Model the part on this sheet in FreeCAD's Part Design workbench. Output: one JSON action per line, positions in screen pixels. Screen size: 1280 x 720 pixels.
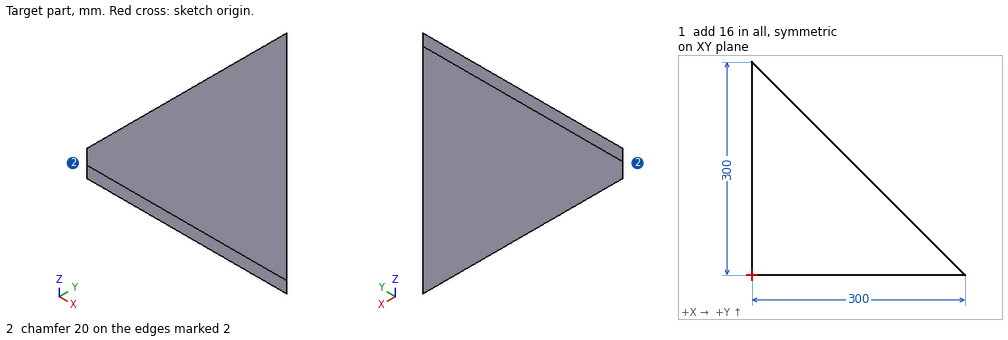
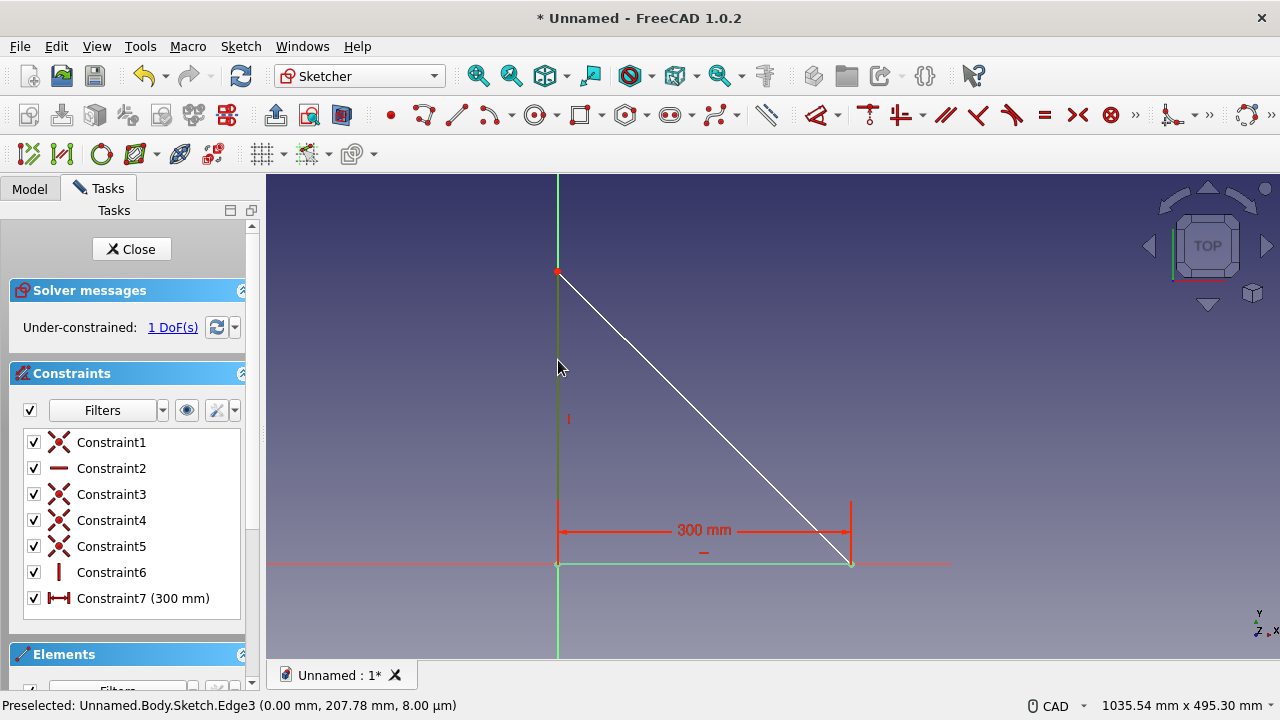
{"action": "key", "text": "i"}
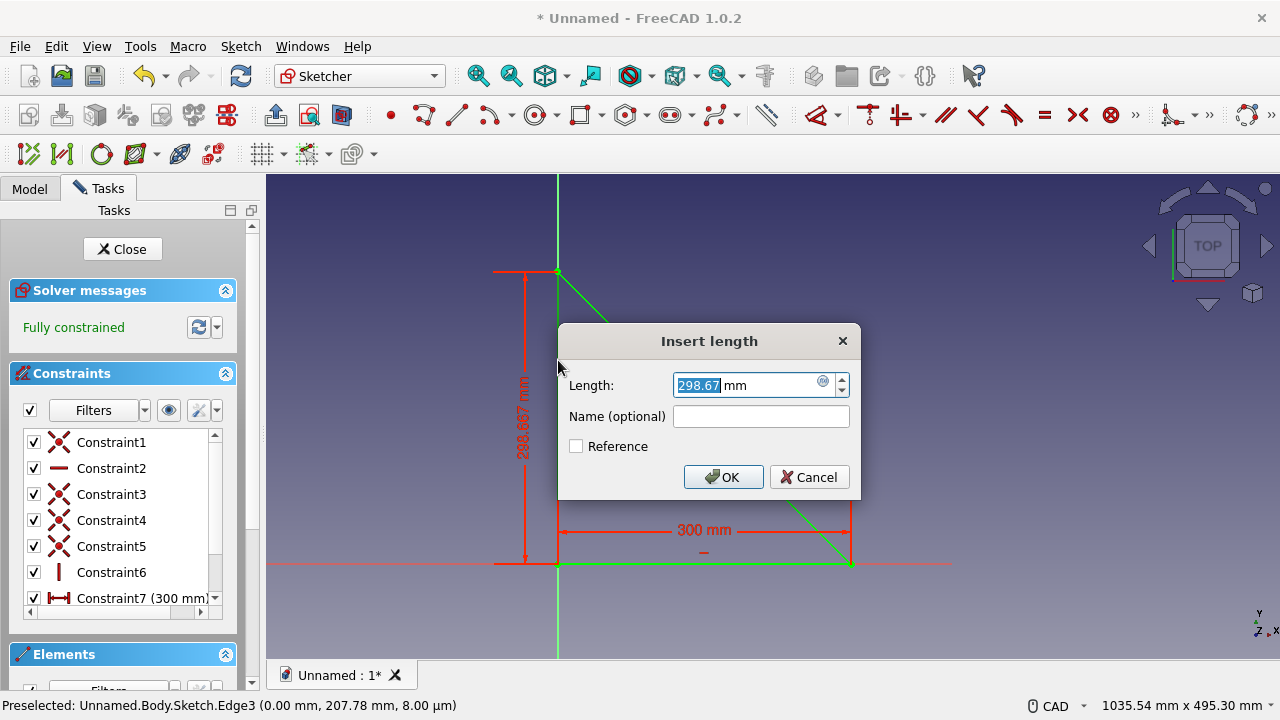
{"action": "type", "text": "300"}
{"action": "key", "text": "Return"}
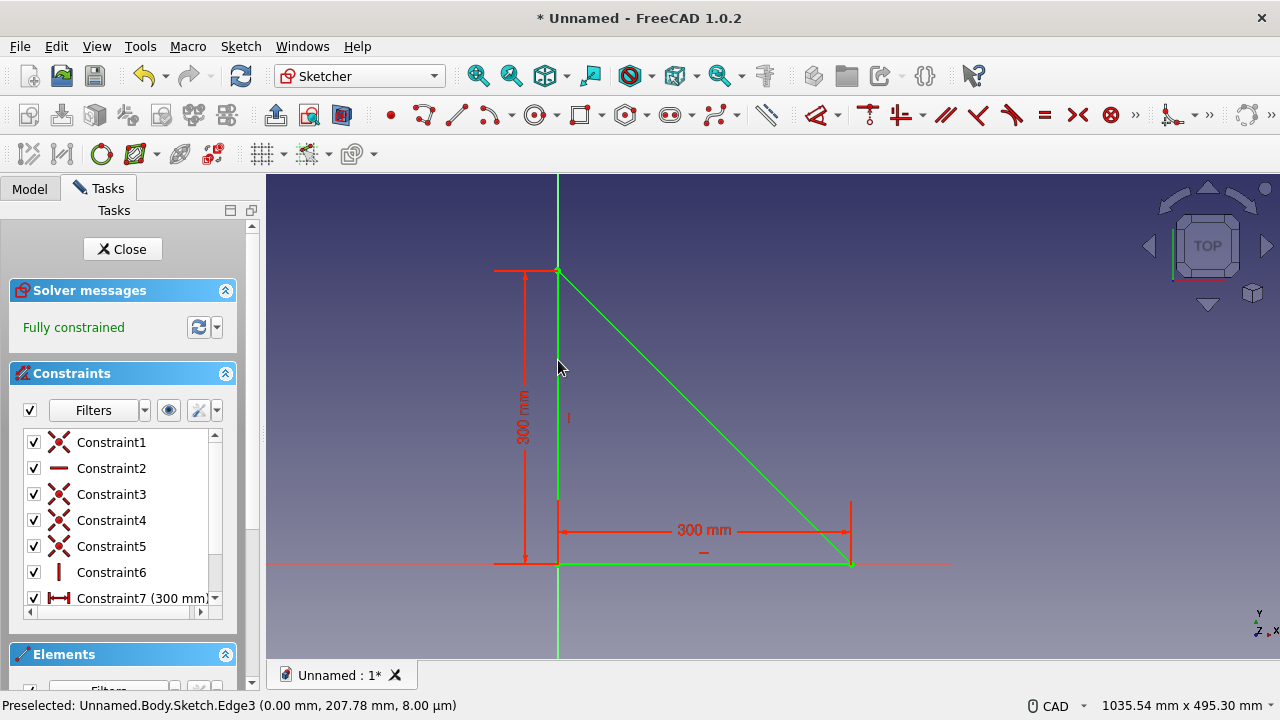
{"action": "left_click", "coordinate": [123, 249]}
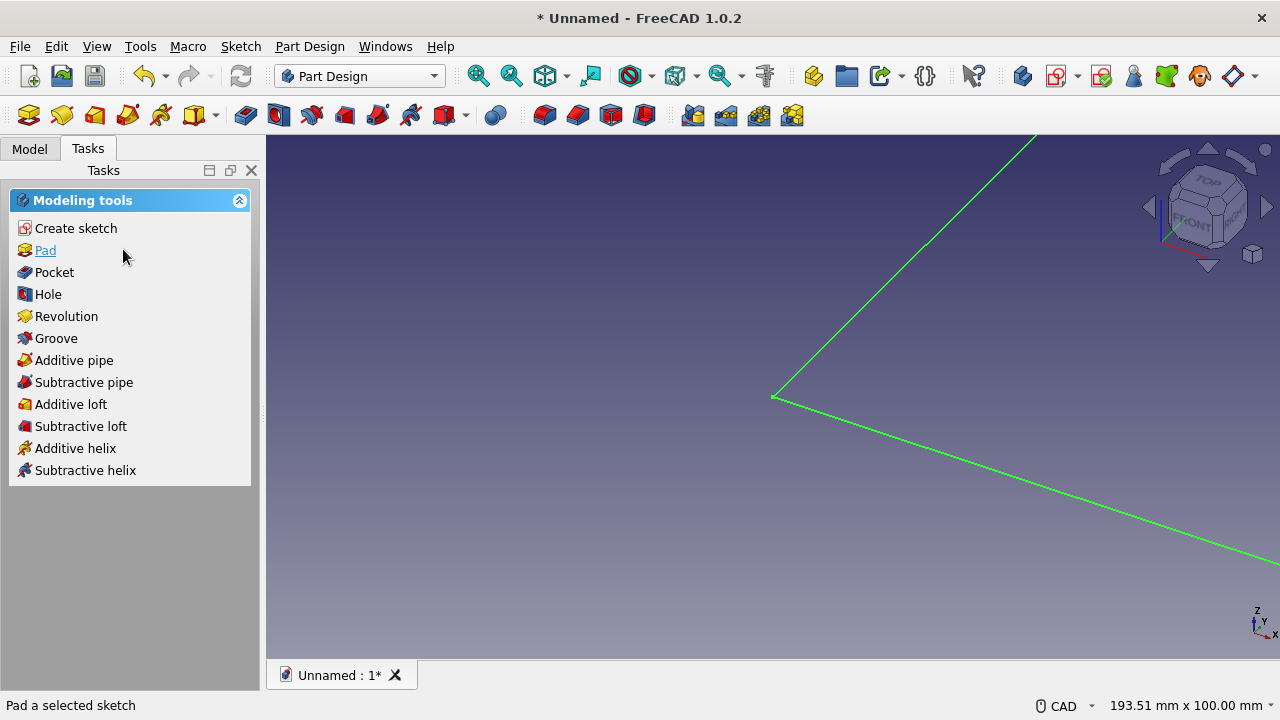
{"action": "left_click", "coordinate": [29, 116]}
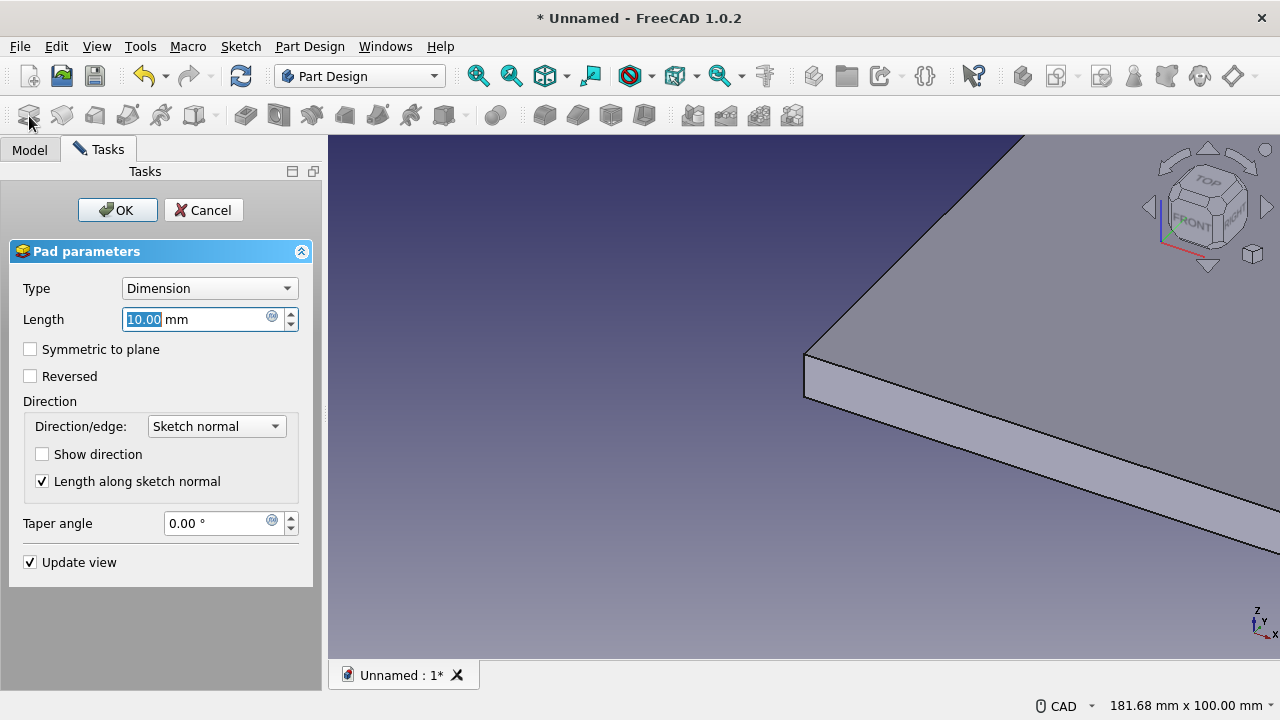
{"action": "type", "text": "16"}
{"action": "key", "text": "Tab"}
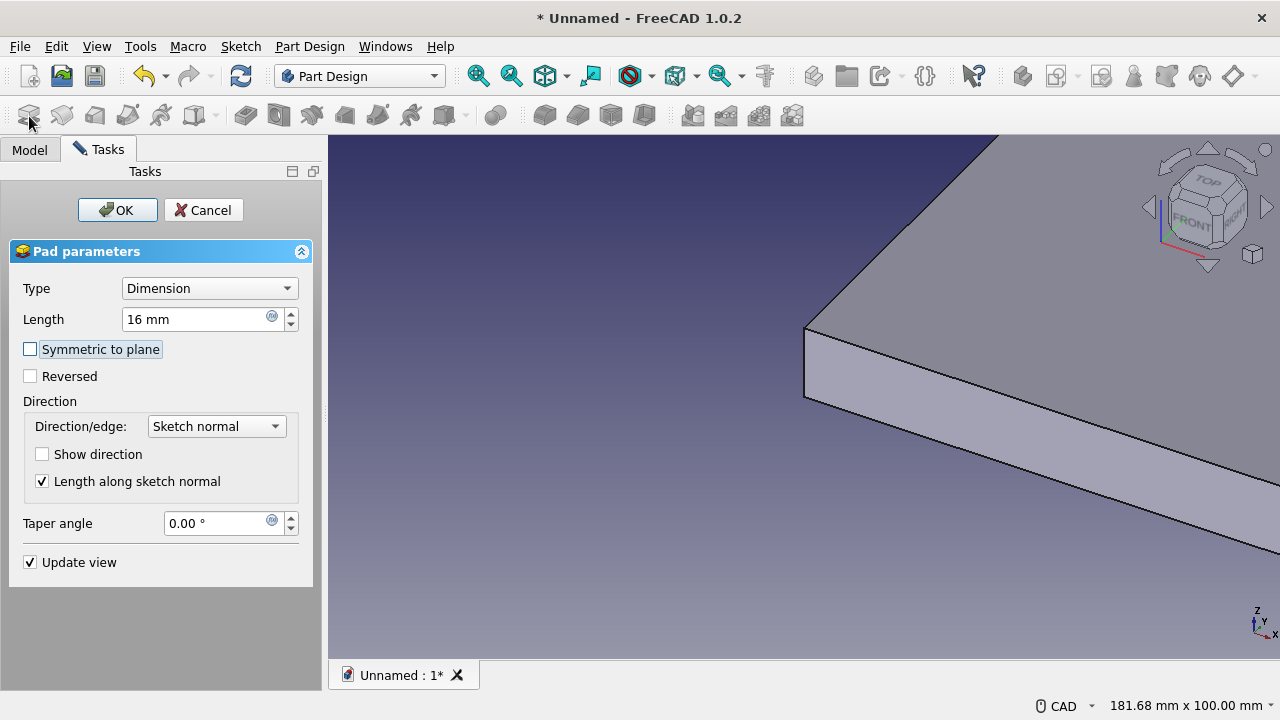
{"action": "left_click", "coordinate": [31, 349]}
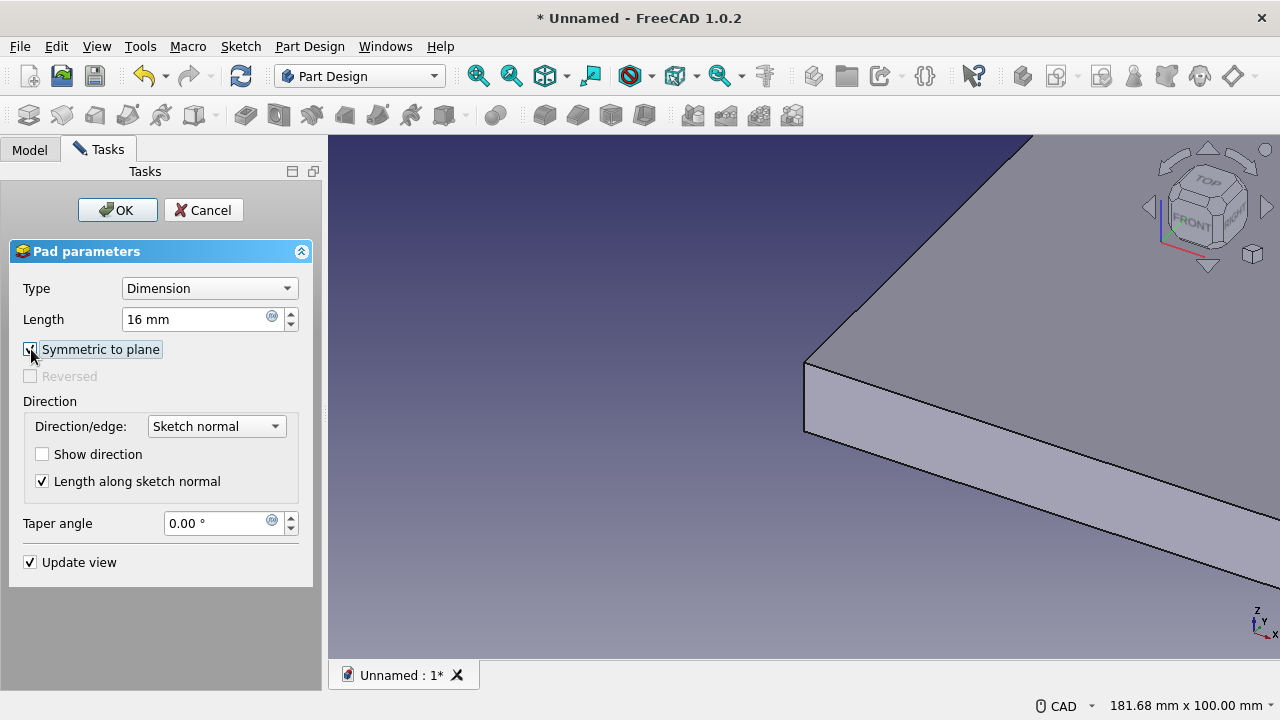
{"action": "left_click", "coordinate": [118, 210]}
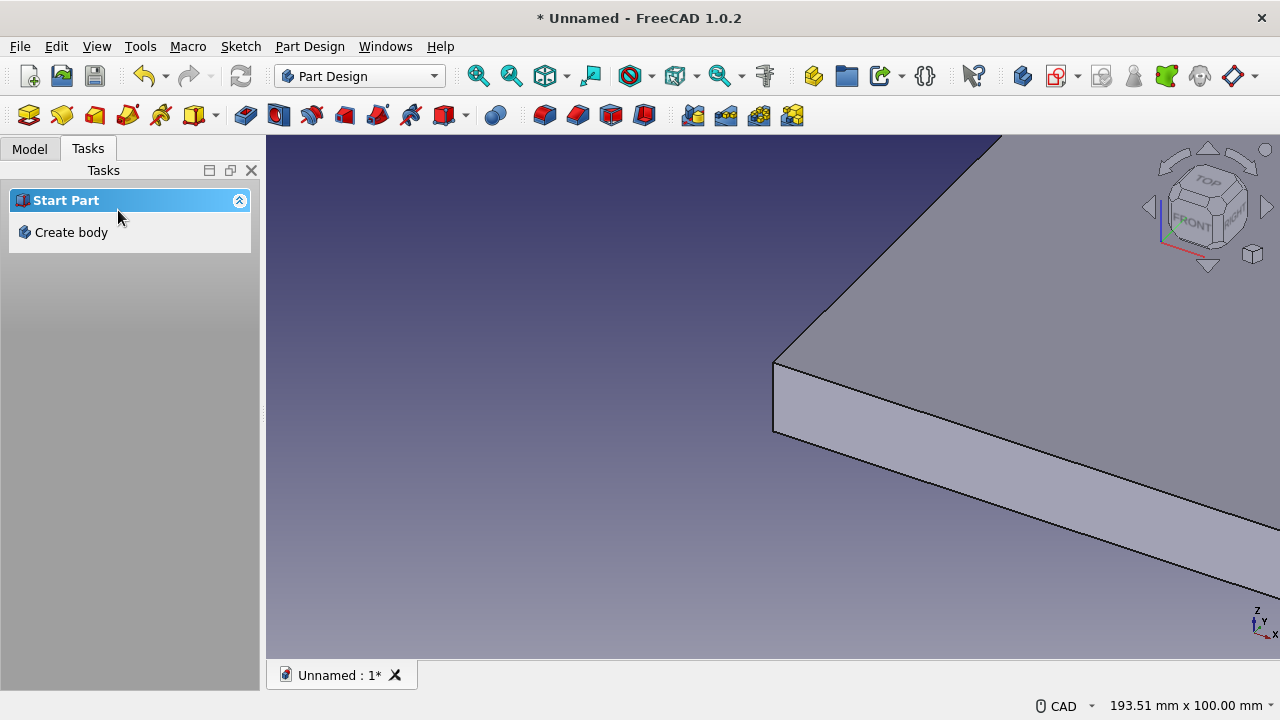
{"action": "left_click", "coordinate": [479, 76]}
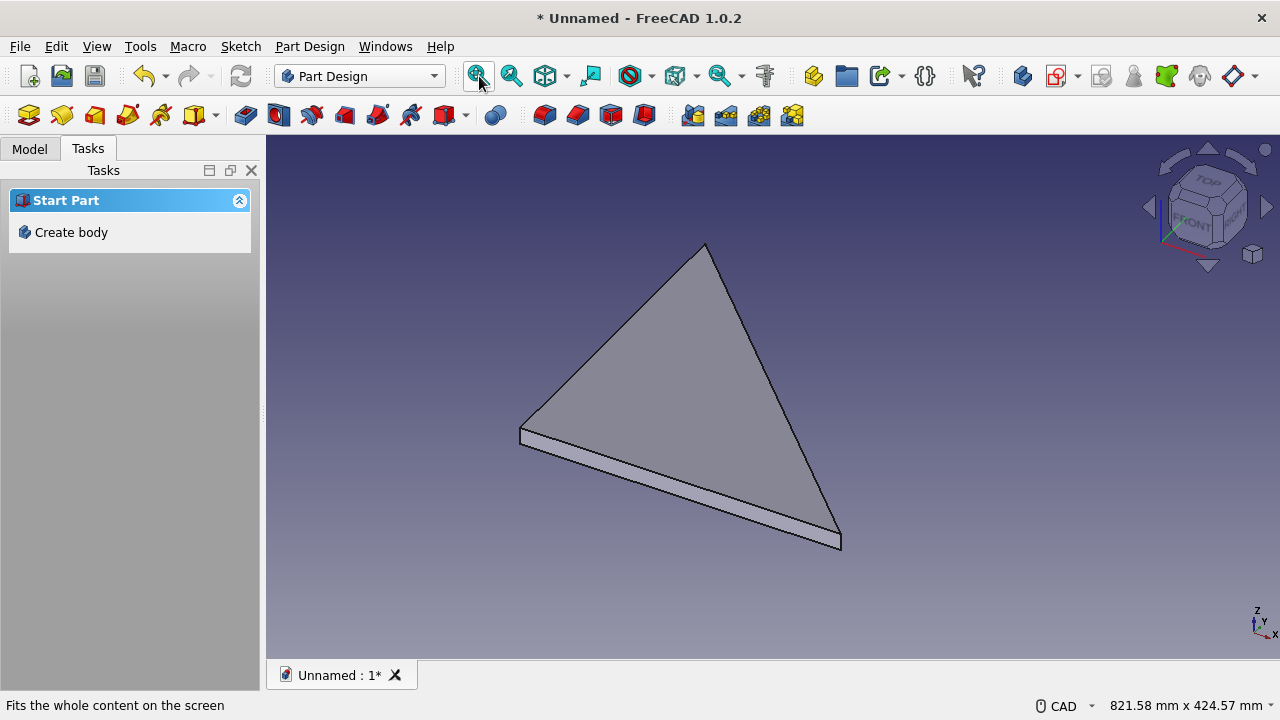
{"action": "scroll", "coordinate": [520, 435], "scroll_direction": "up", "scroll_amount": 4}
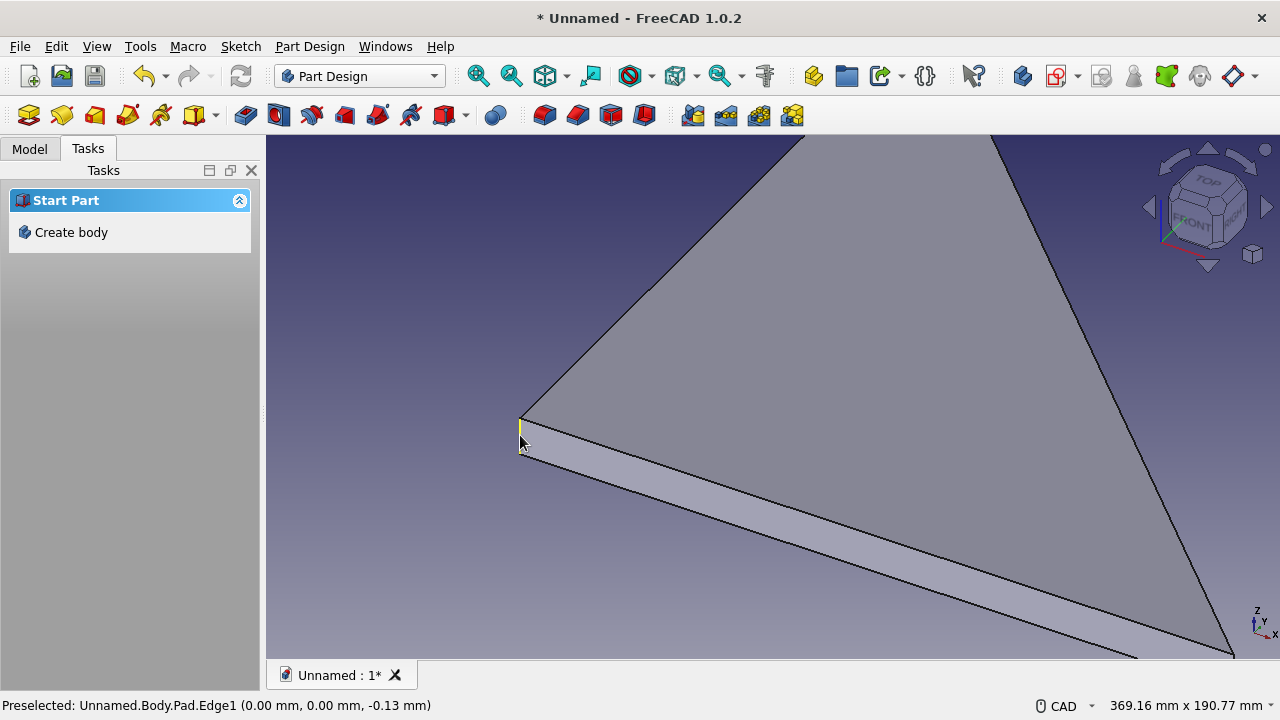
{"action": "left_click", "coordinate": [479, 76]}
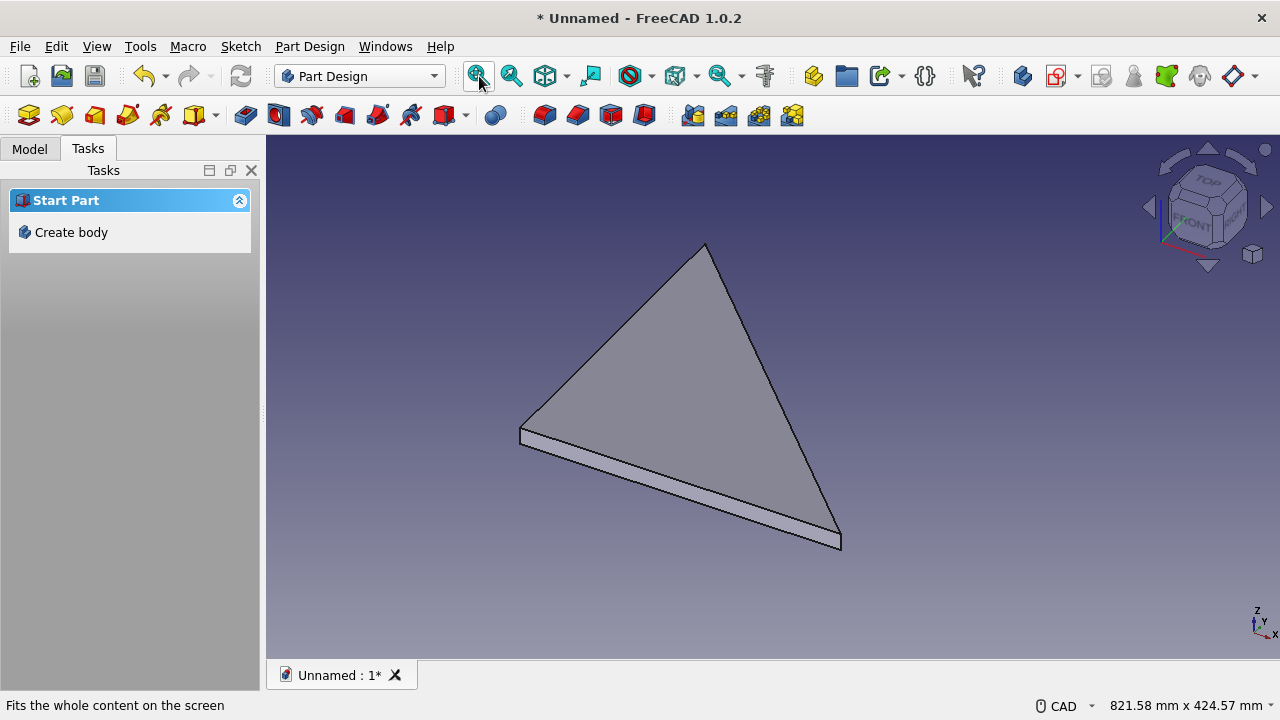
{"action": "key", "text": "0"}